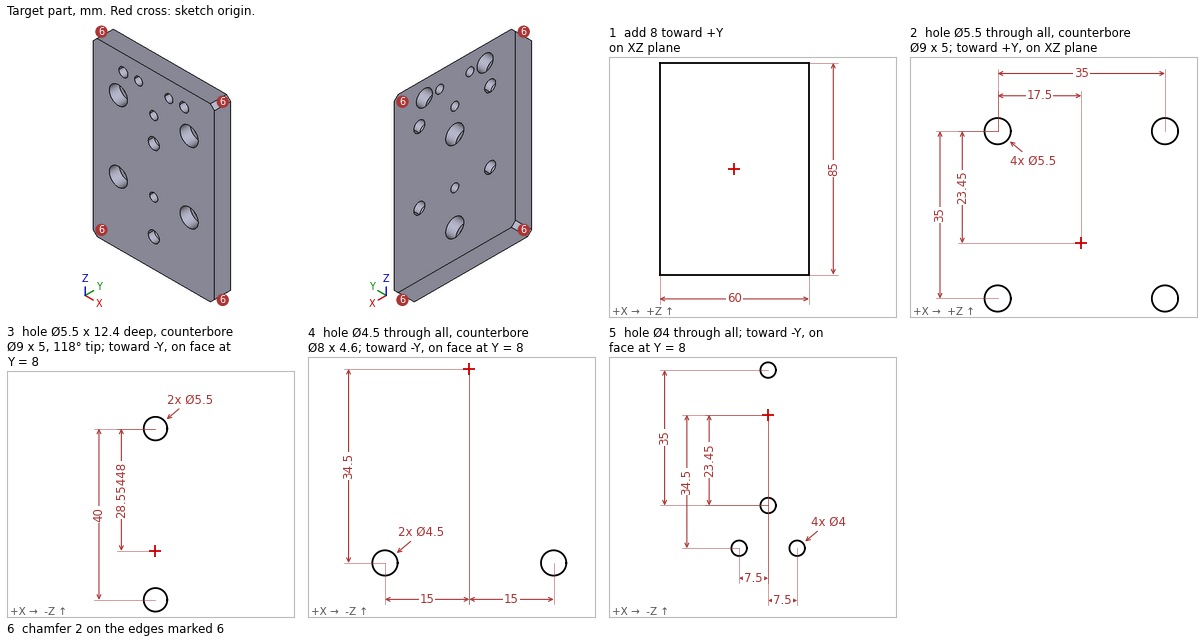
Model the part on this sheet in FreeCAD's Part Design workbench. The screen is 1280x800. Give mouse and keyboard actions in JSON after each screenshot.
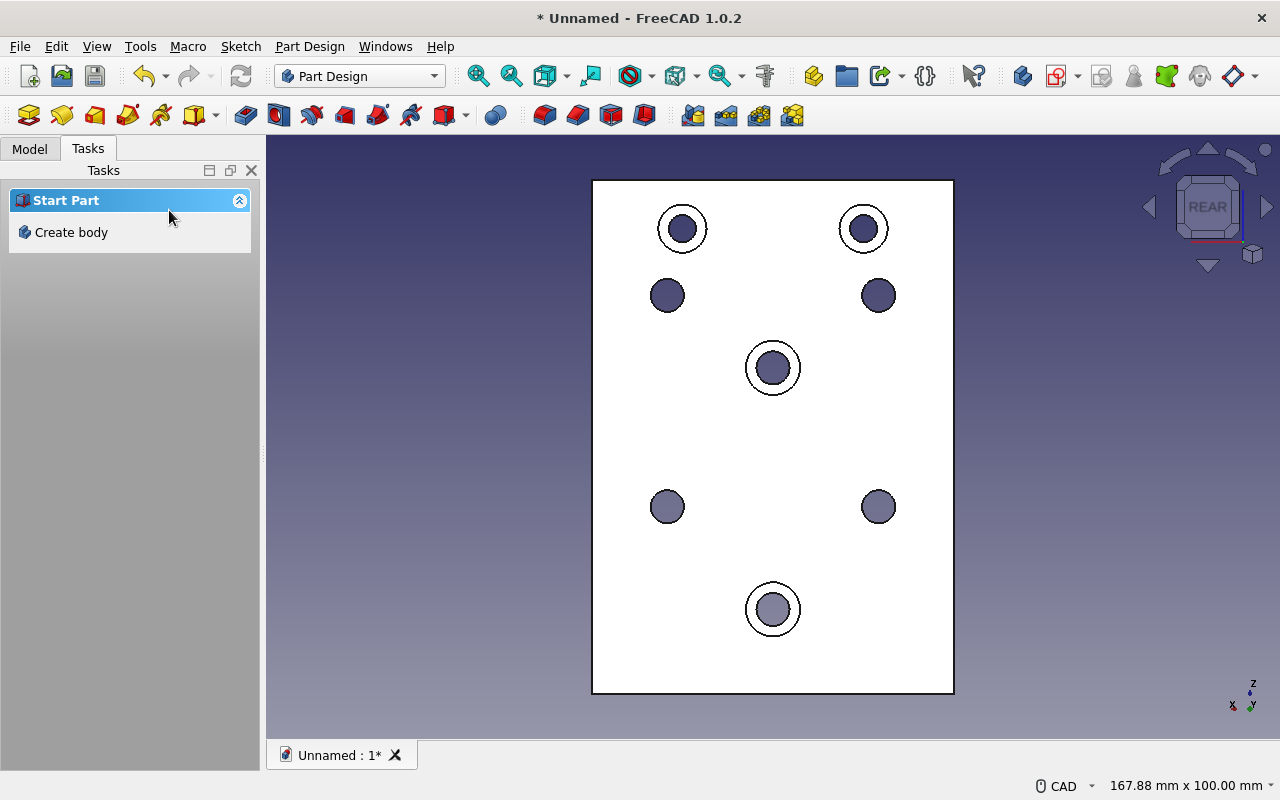
{"action": "left_click", "coordinate": [773, 509]}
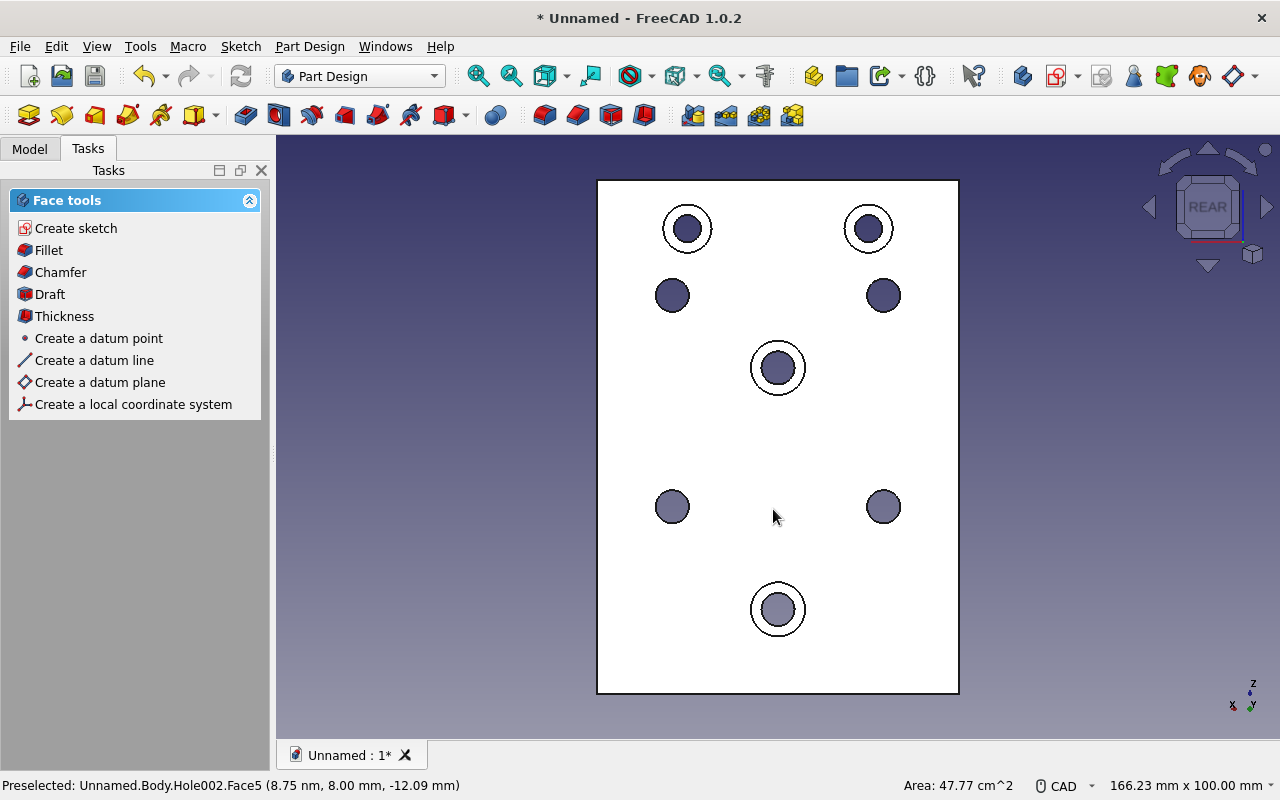
{"action": "left_click", "coordinate": [1056, 76]}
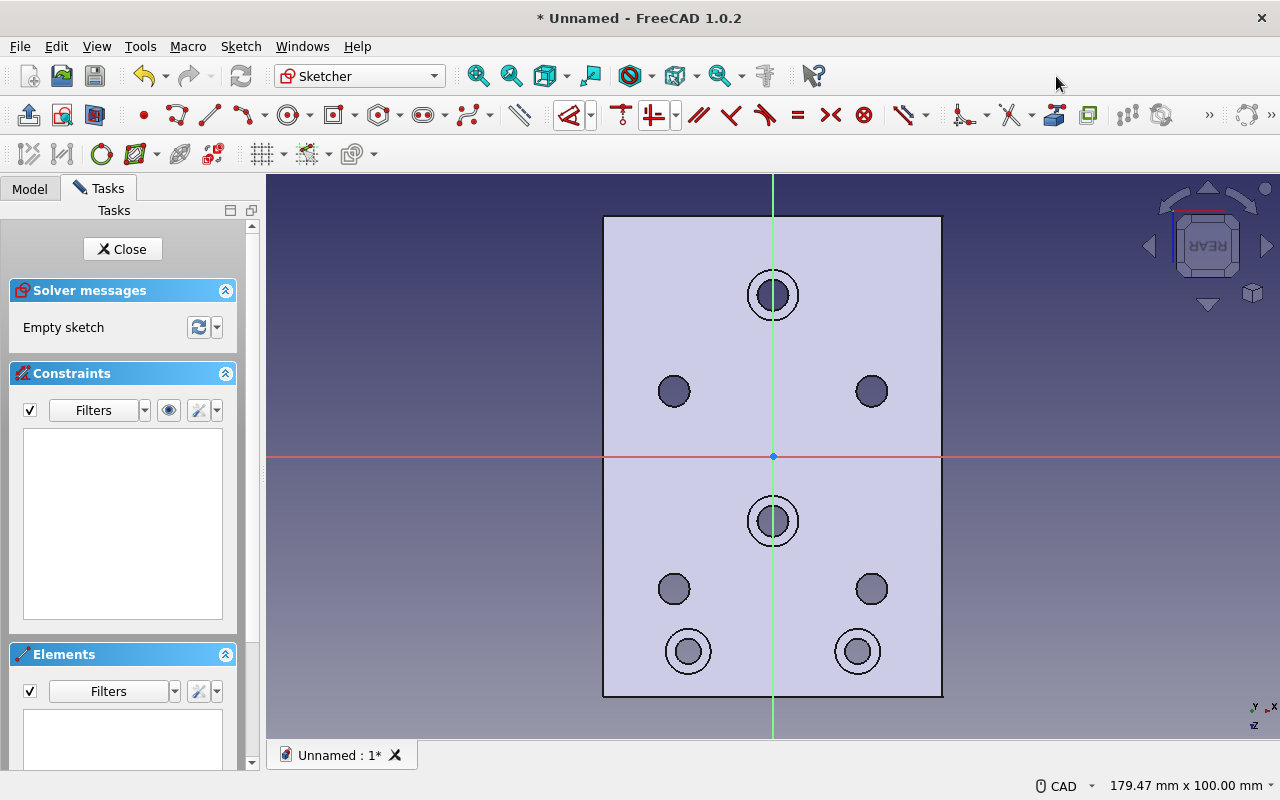
{"action": "left_click", "coordinate": [288, 116]}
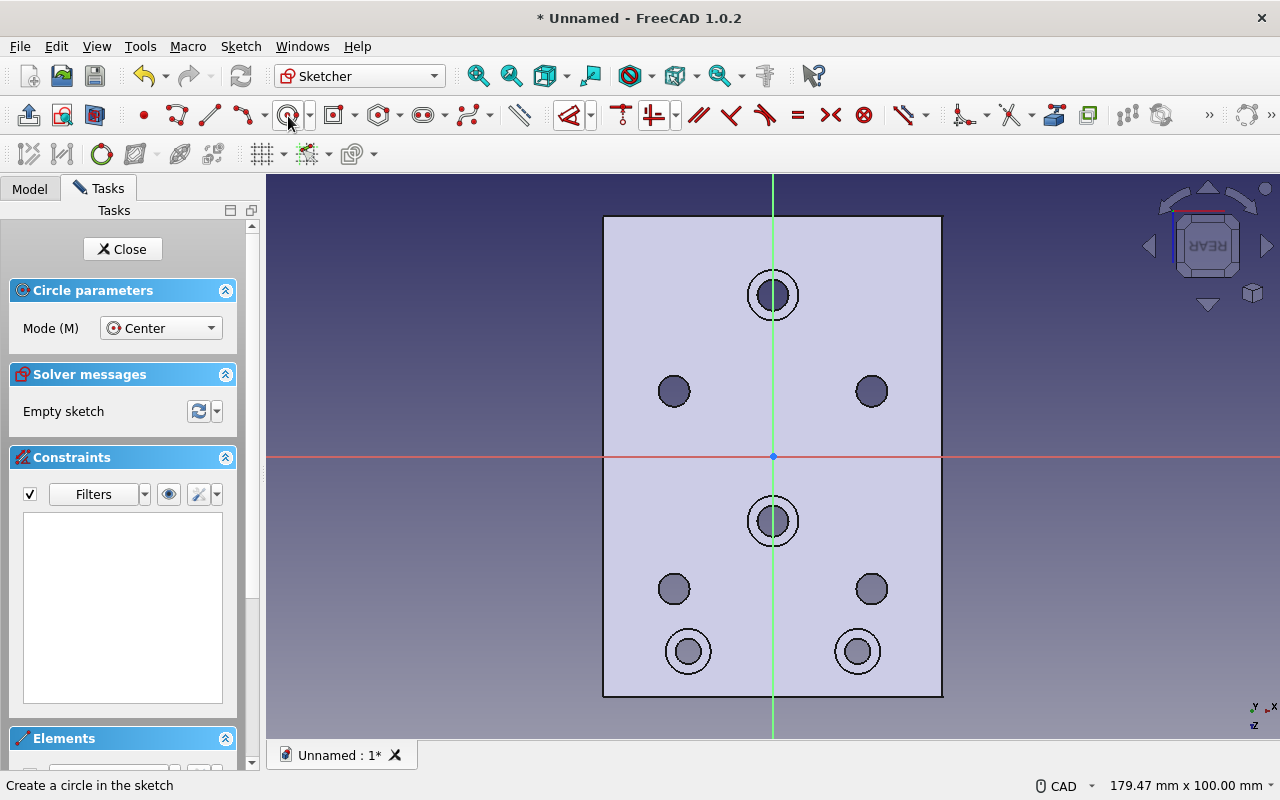
{"action": "scroll", "coordinate": [731, 651], "scroll_direction": "up", "scroll_amount": 4}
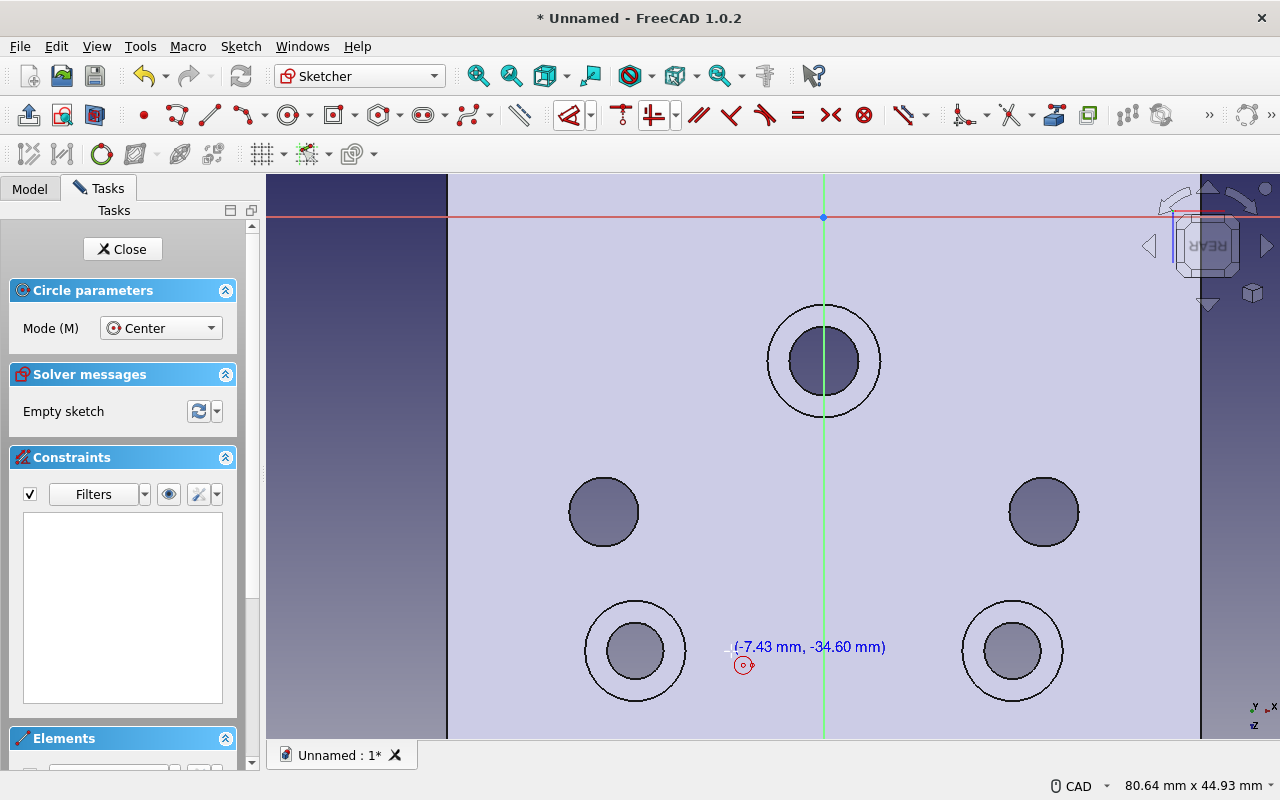
{"action": "left_click", "coordinate": [730, 651]}
{"action": "left_click", "coordinate": [747, 633]}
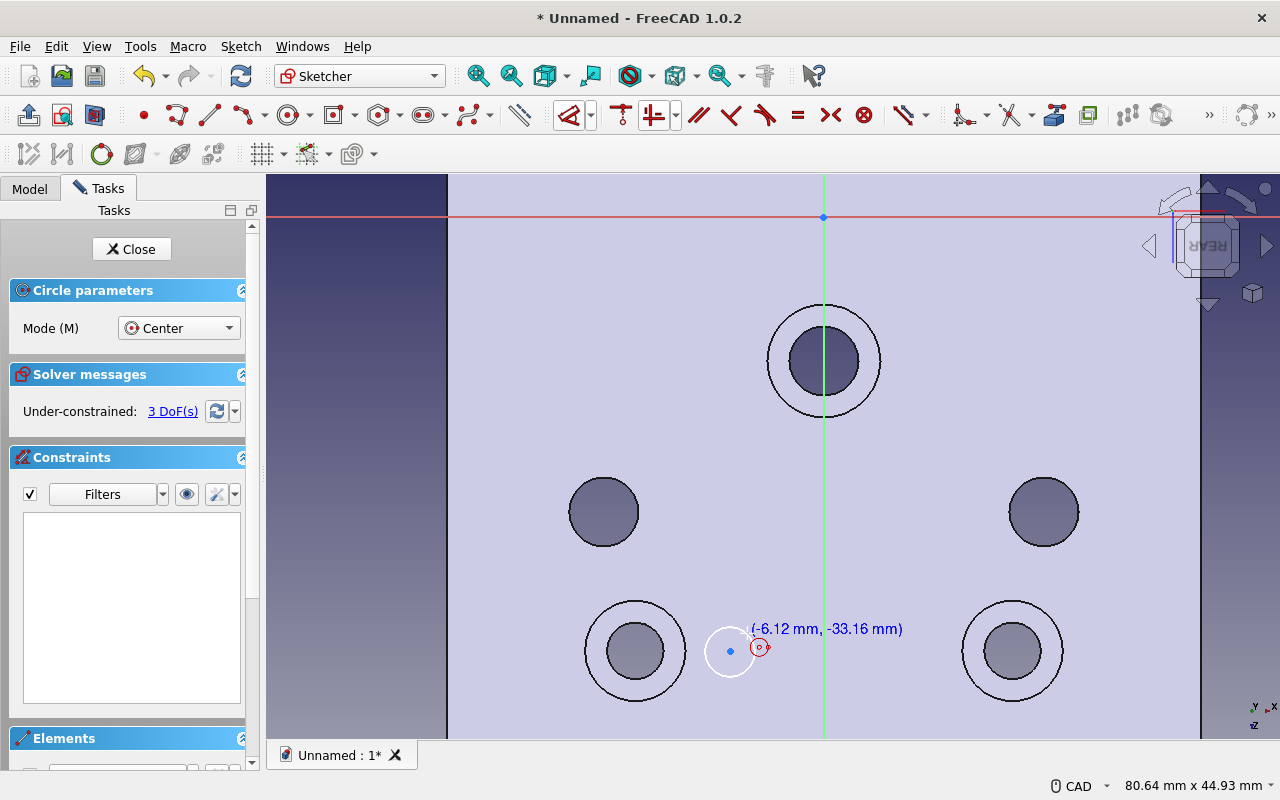
{"action": "left_click", "coordinate": [918, 651]}
{"action": "left_click", "coordinate": [936, 633]}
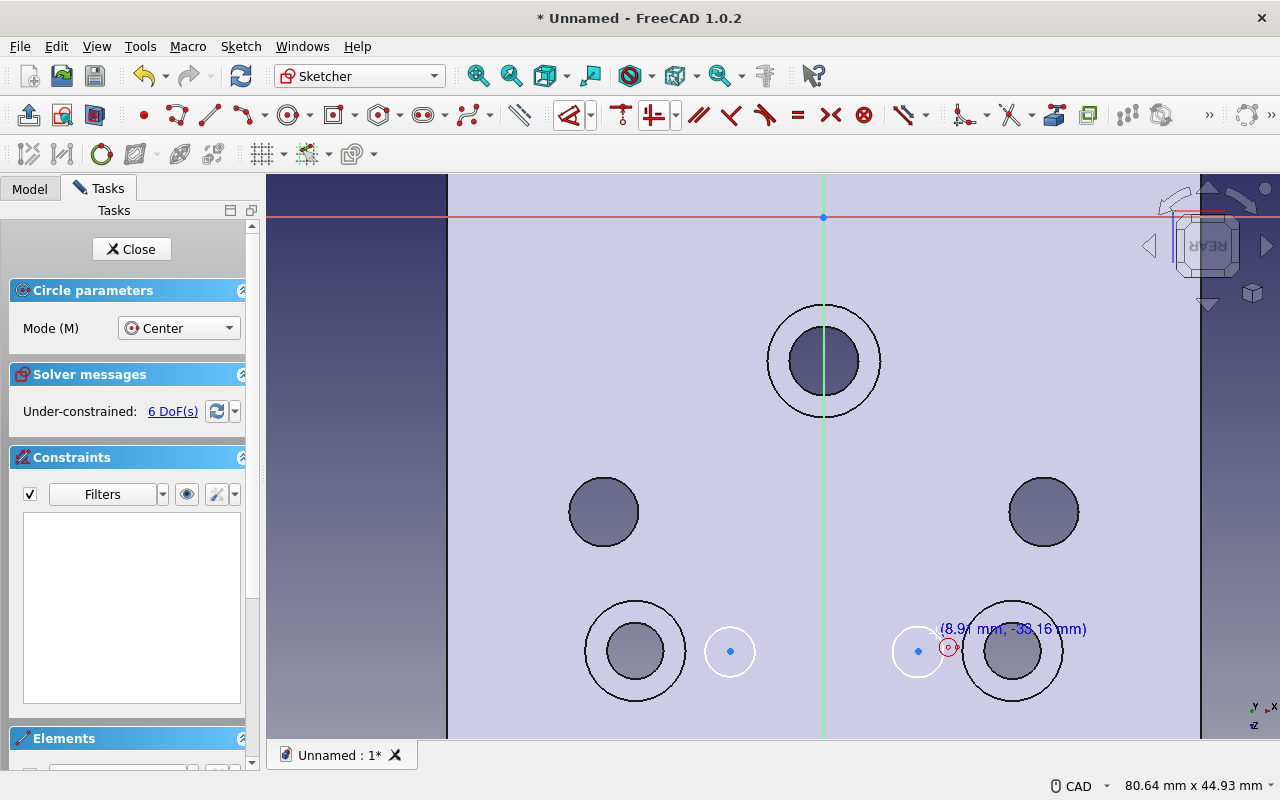
{"action": "left_click", "coordinate": [824, 512]}
{"action": "left_click", "coordinate": [842, 494]}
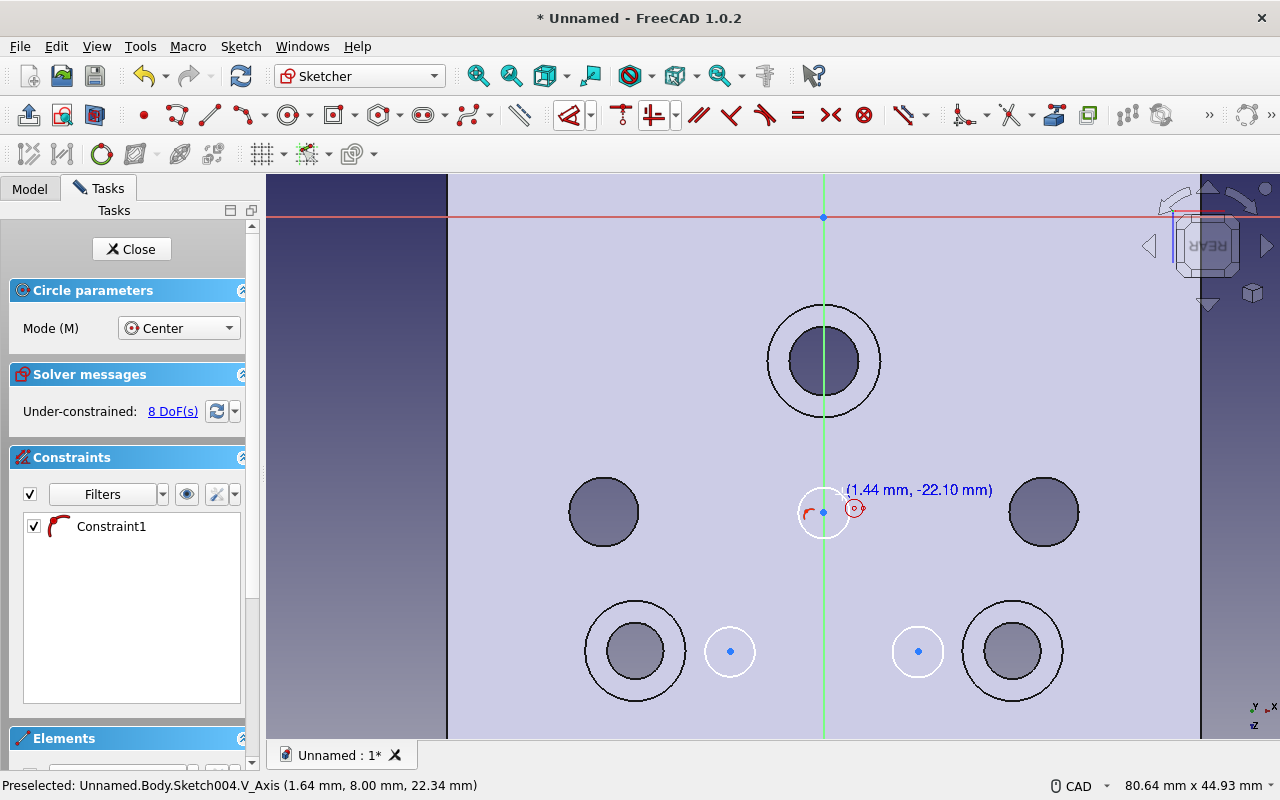
{"action": "scroll", "coordinate": [559, 572], "scroll_direction": "down", "scroll_amount": 3}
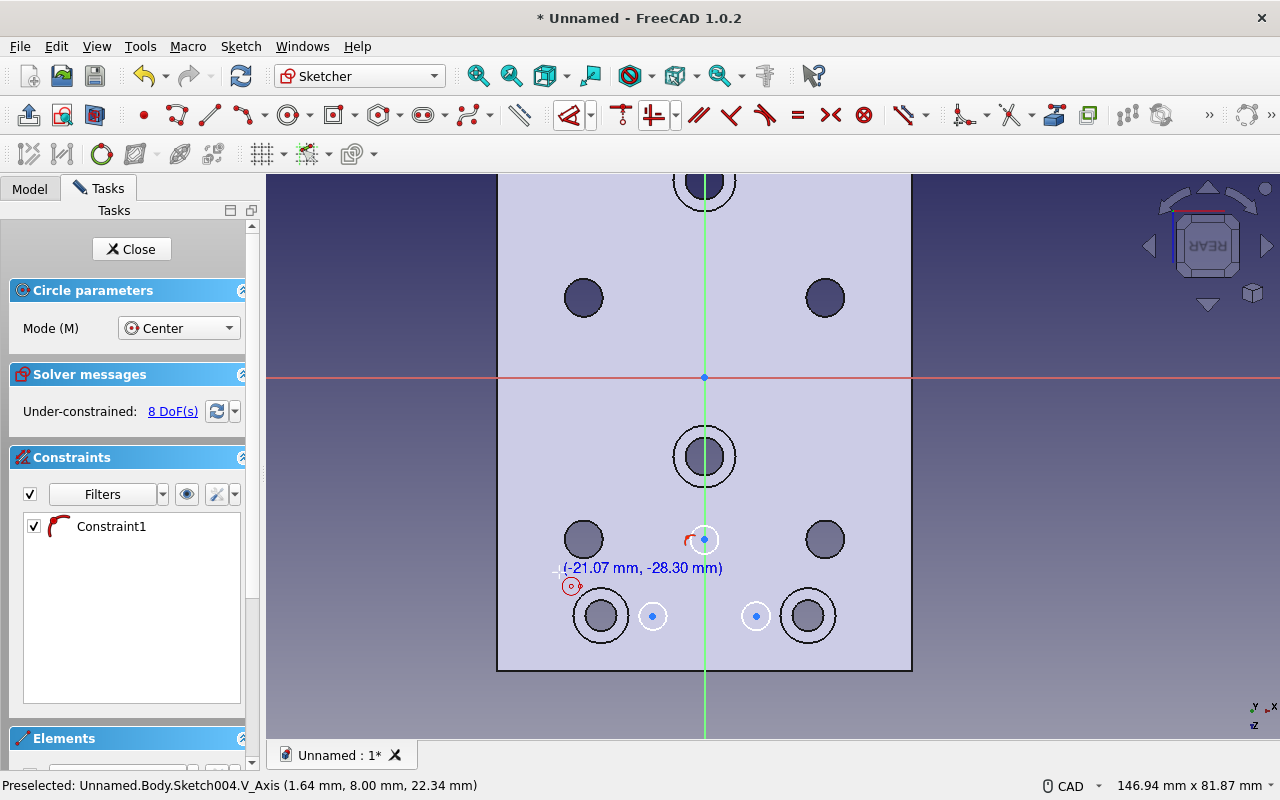
{"action": "scroll", "coordinate": [705, 298], "scroll_direction": "up", "scroll_amount": 3}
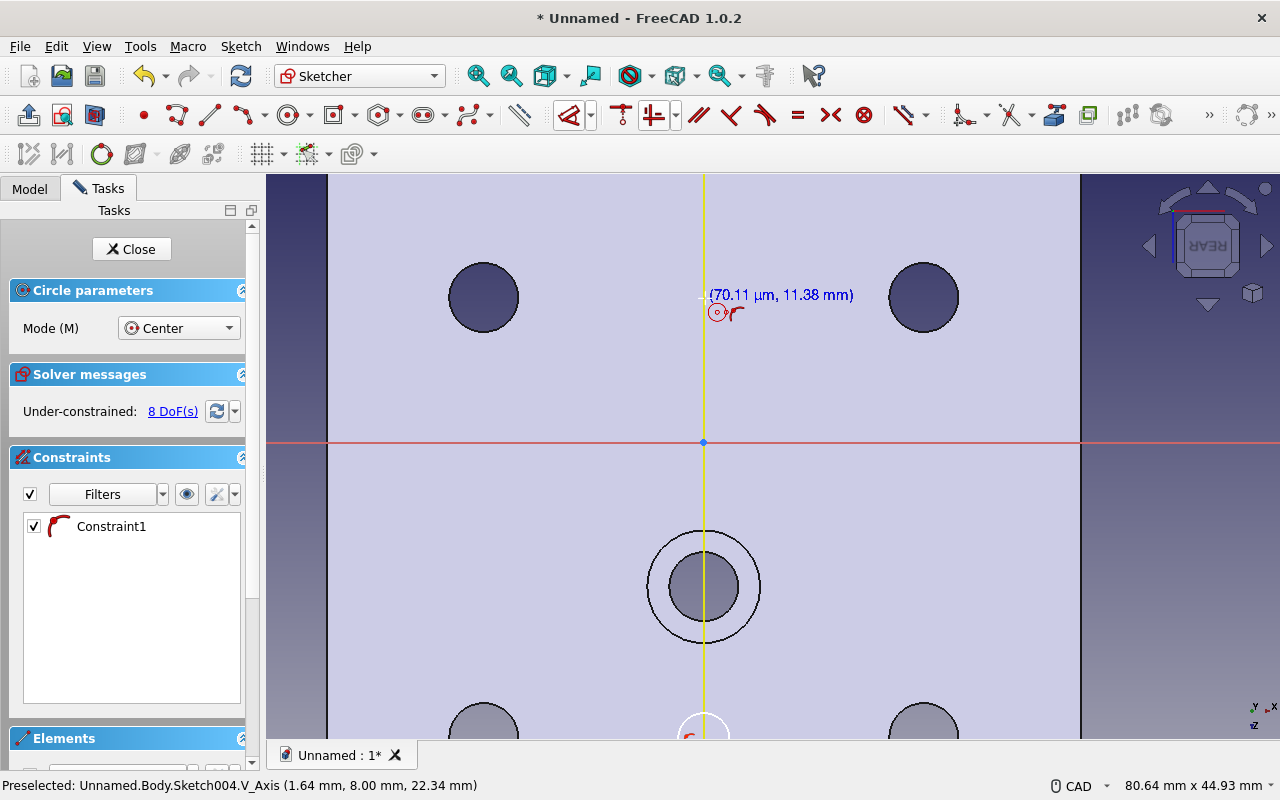
{"action": "left_click", "coordinate": [704, 298]}
{"action": "left_click", "coordinate": [722, 280]}
{"action": "key", "text": "Escape"}